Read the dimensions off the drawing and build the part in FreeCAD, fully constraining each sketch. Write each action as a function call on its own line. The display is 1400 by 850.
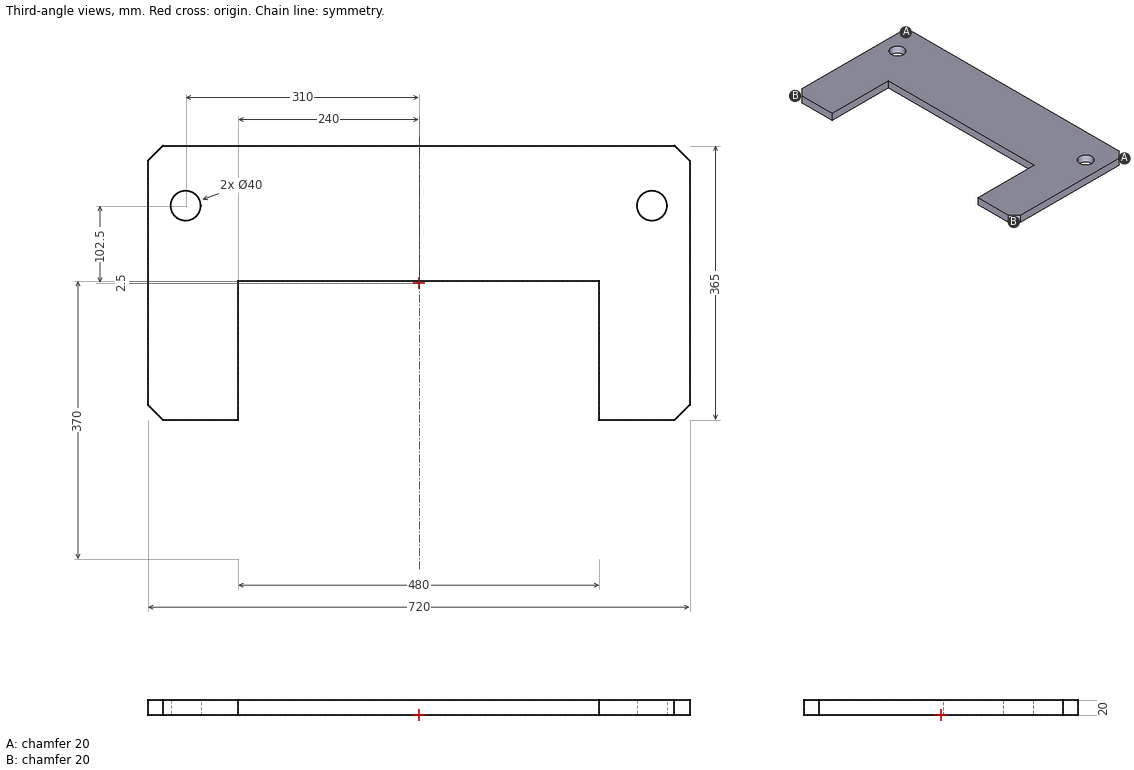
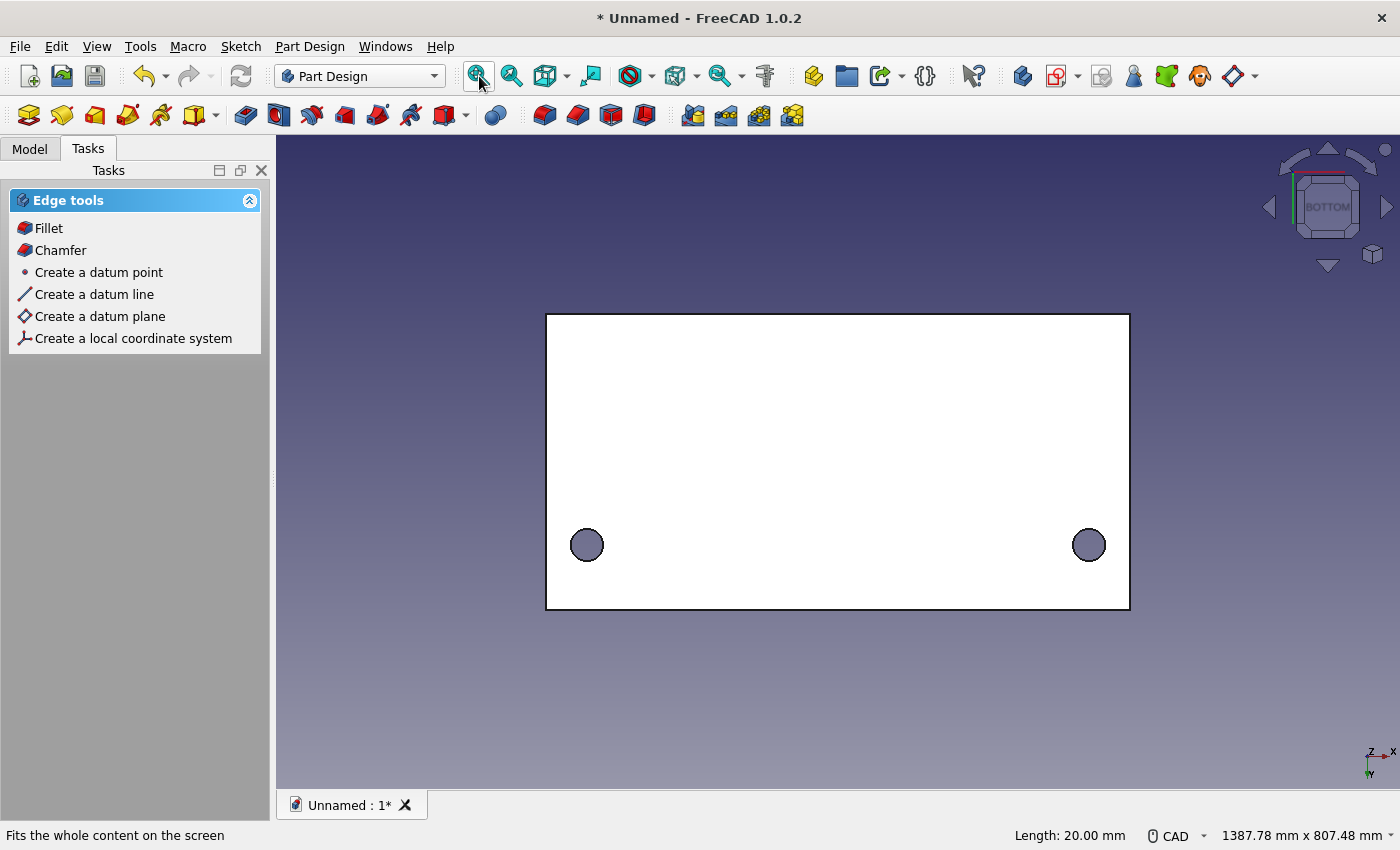
scroll(546, 609, up, 5)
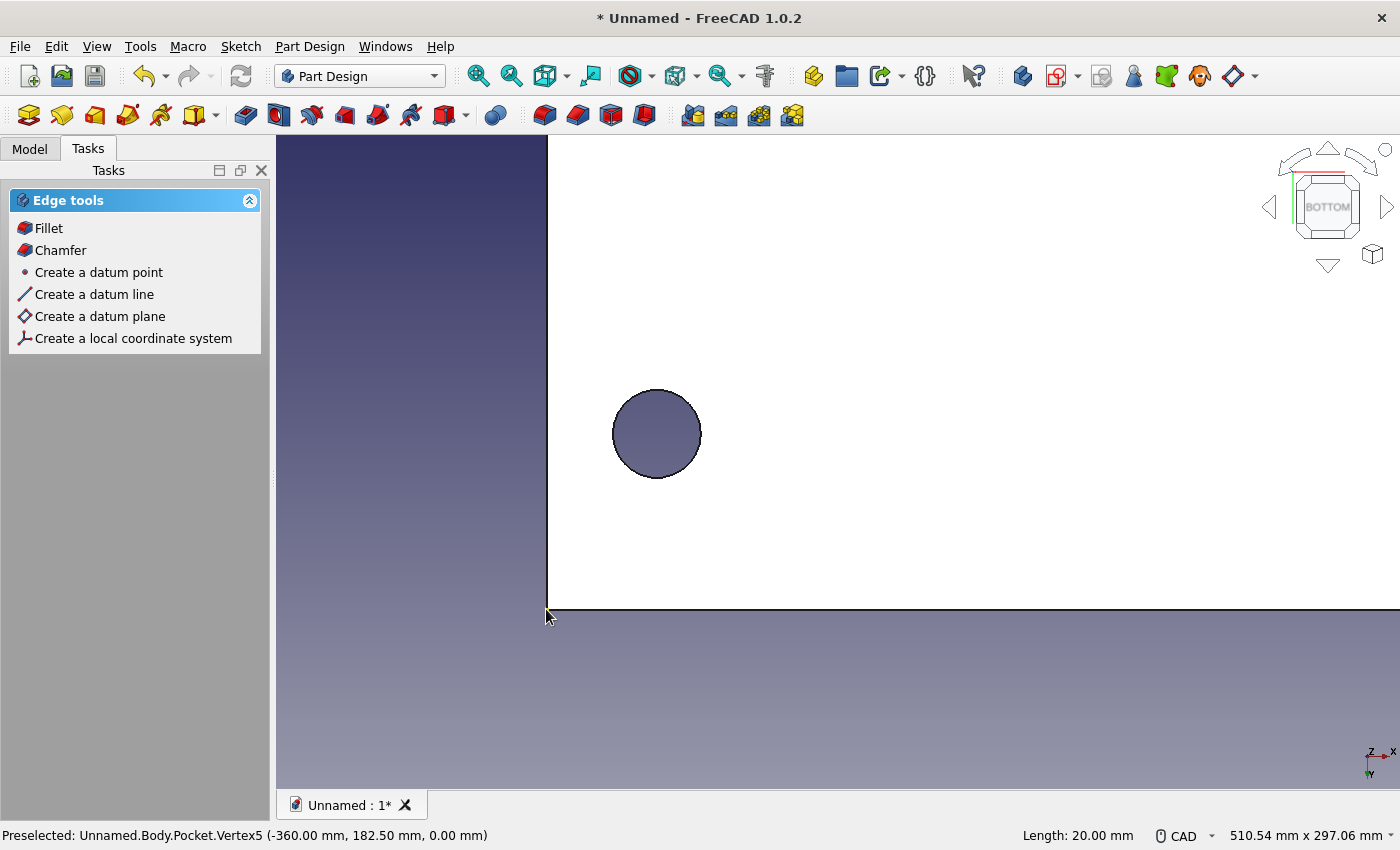
click(479, 76)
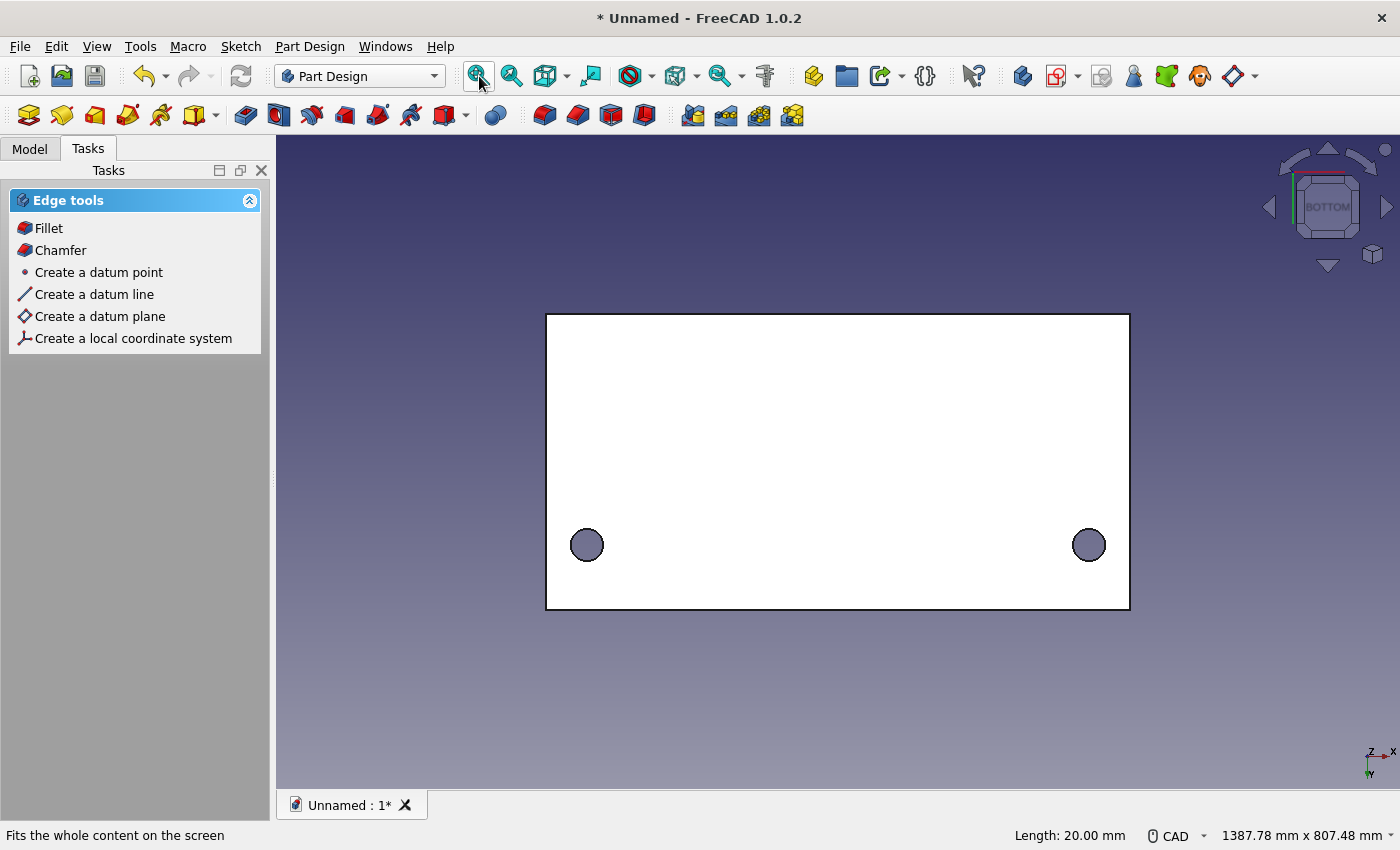
key(4)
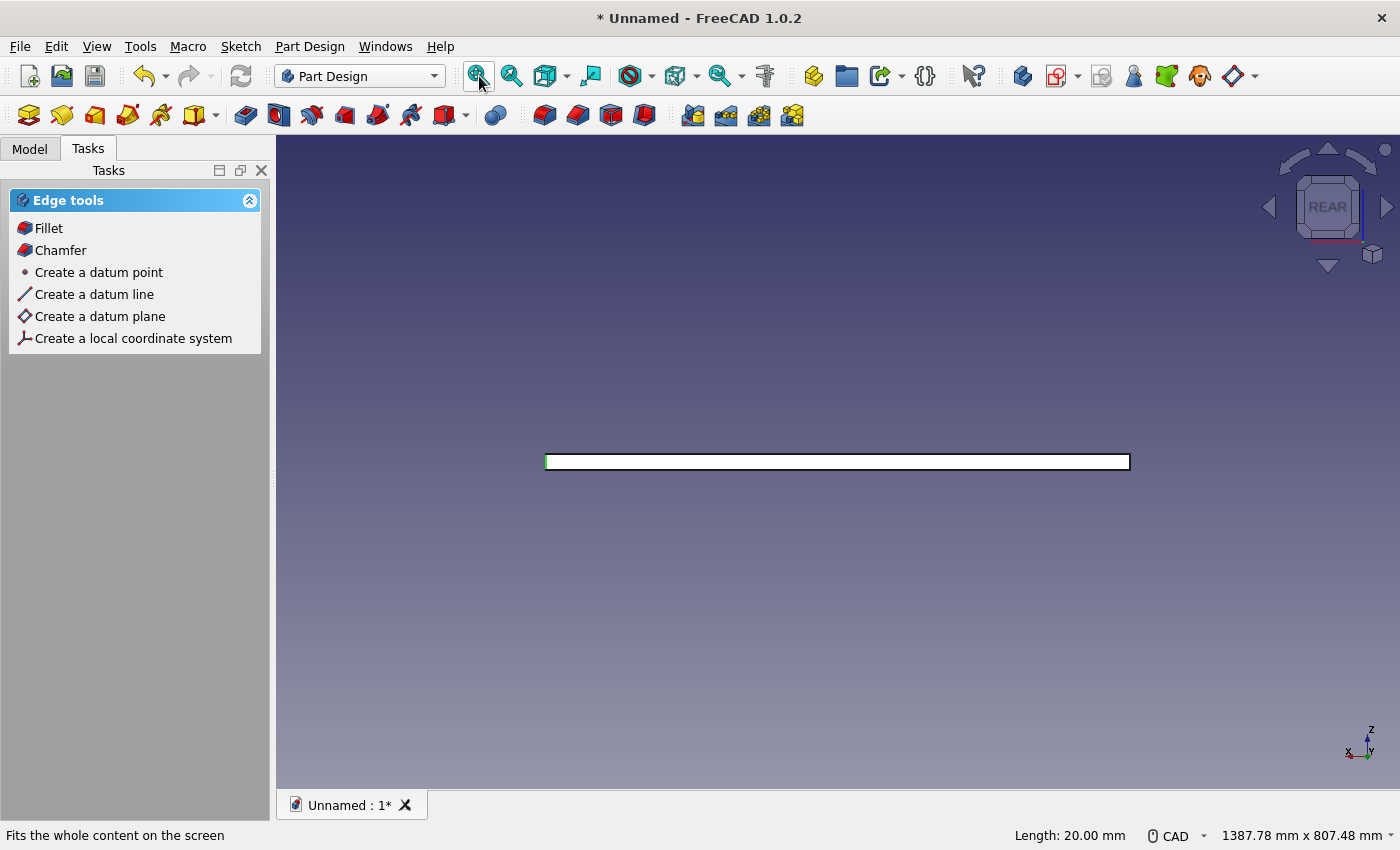
click(1130, 461, ctrl)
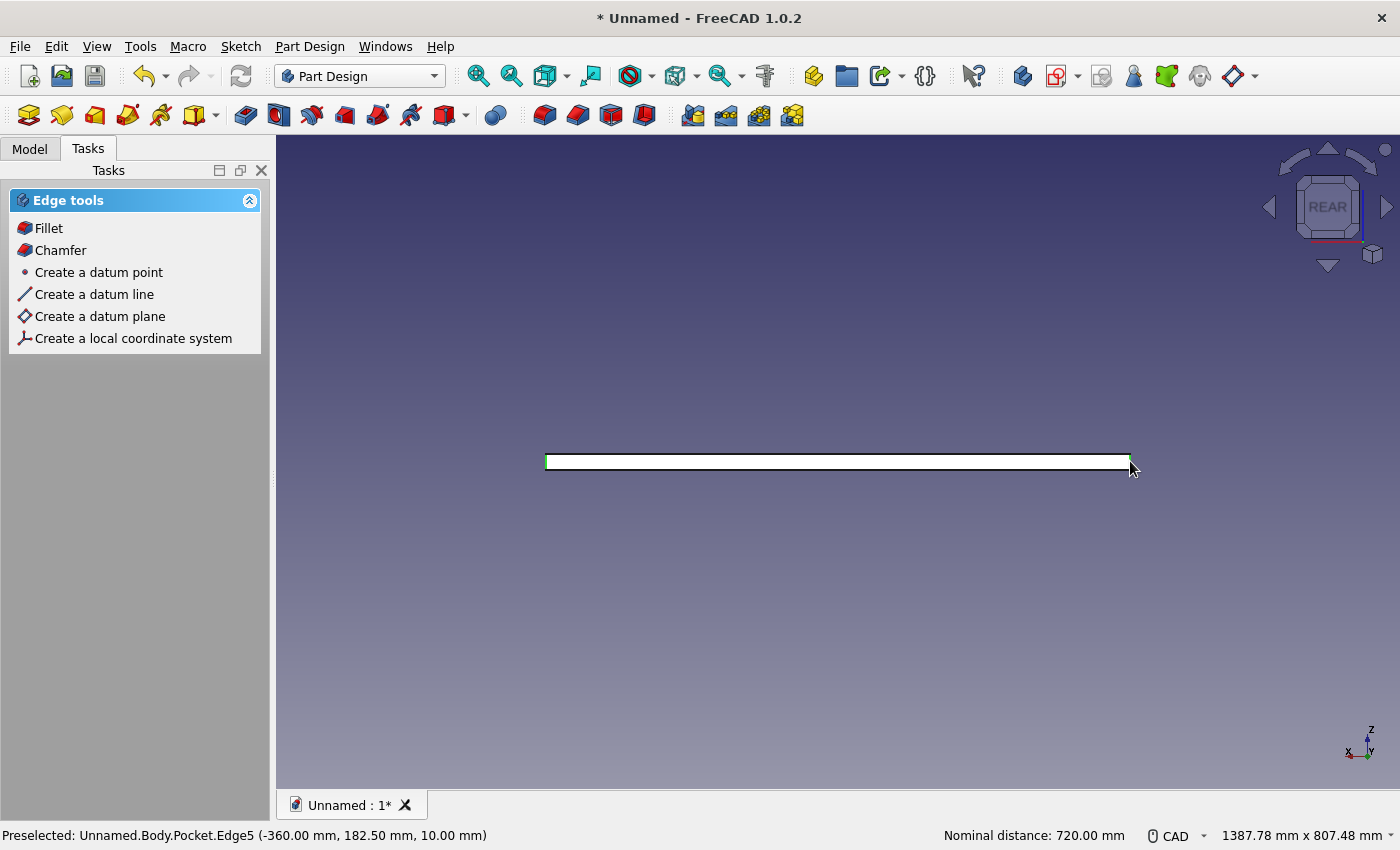
click(578, 116)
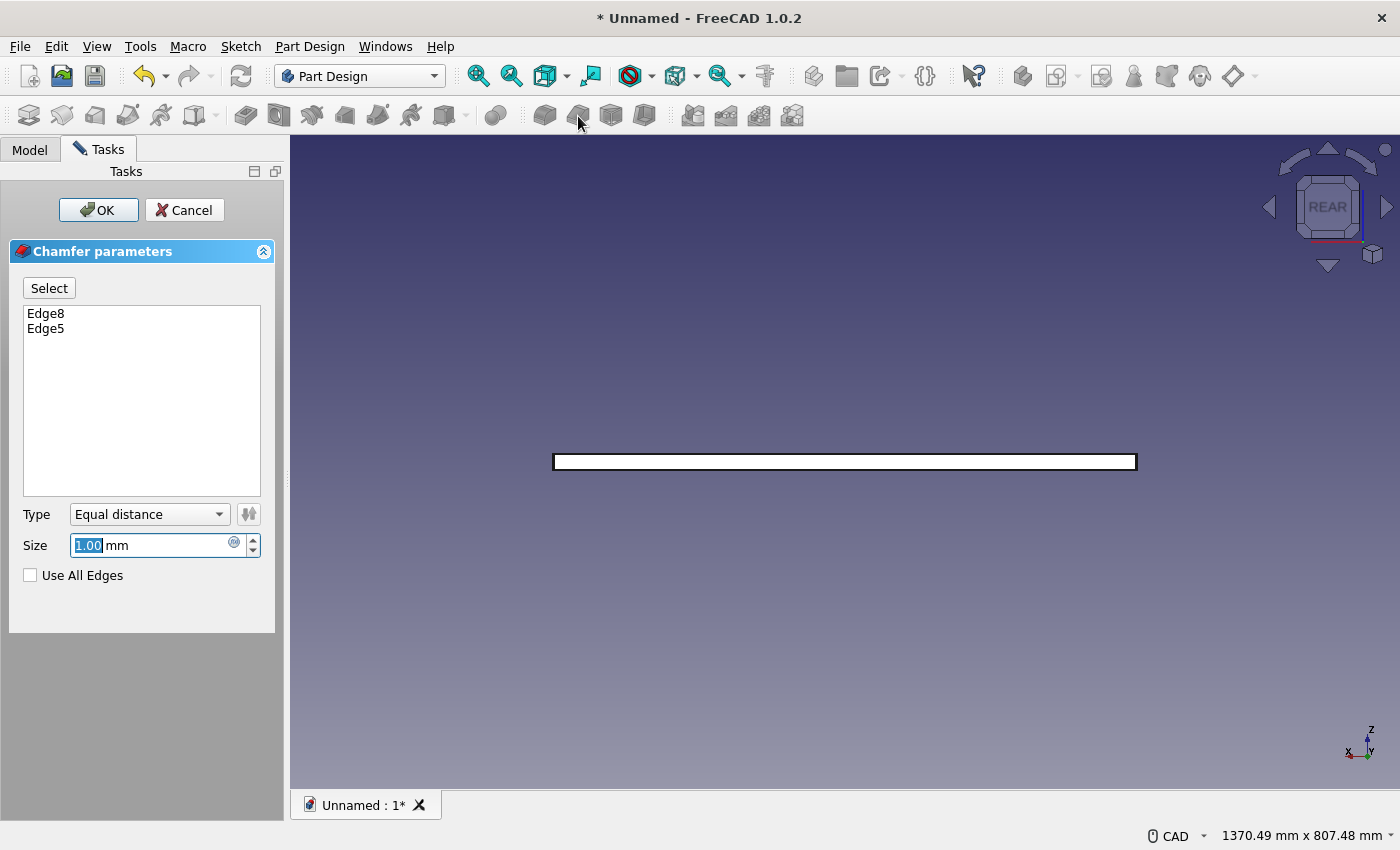
text(20)
key(Tab)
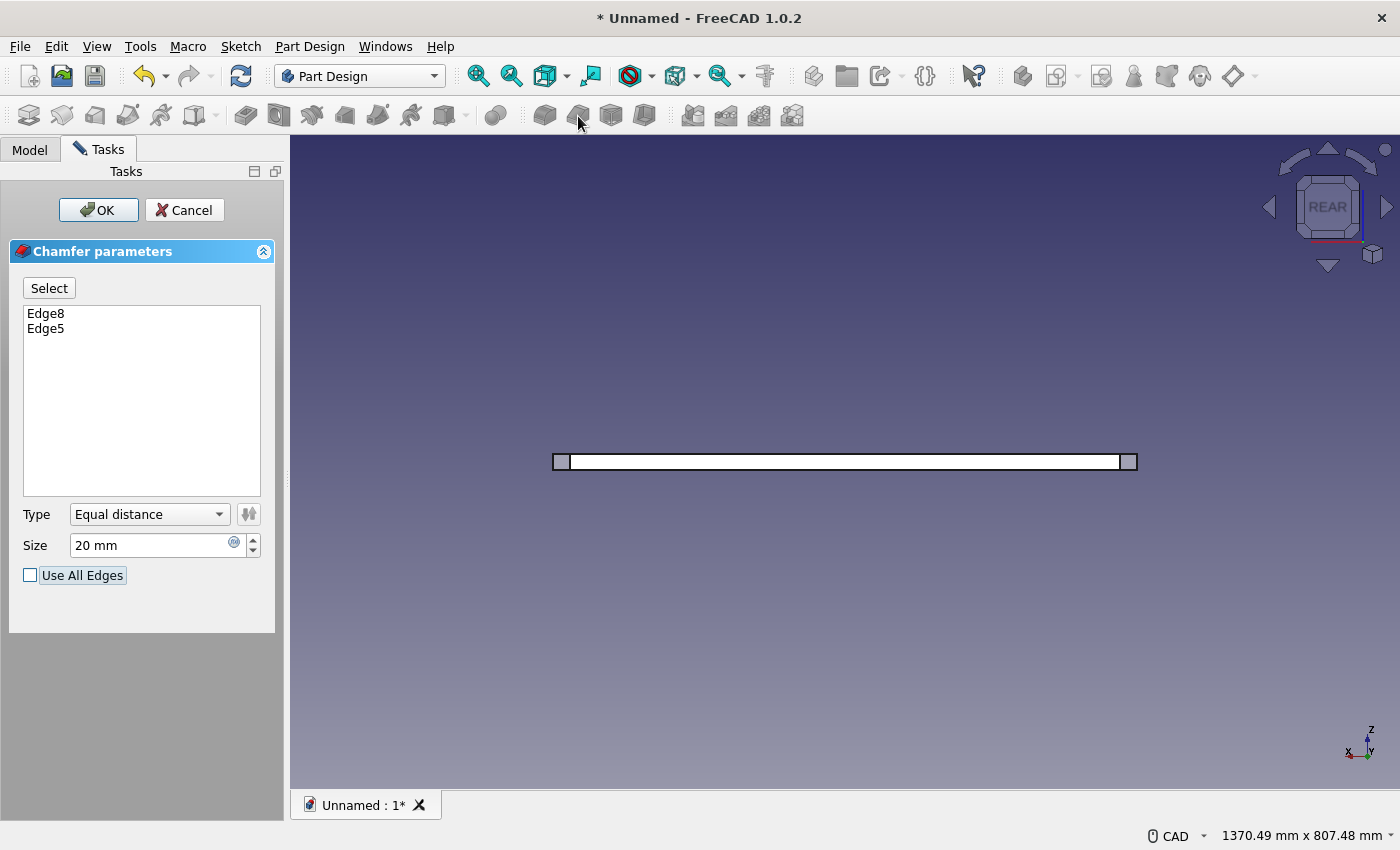
click(99, 210)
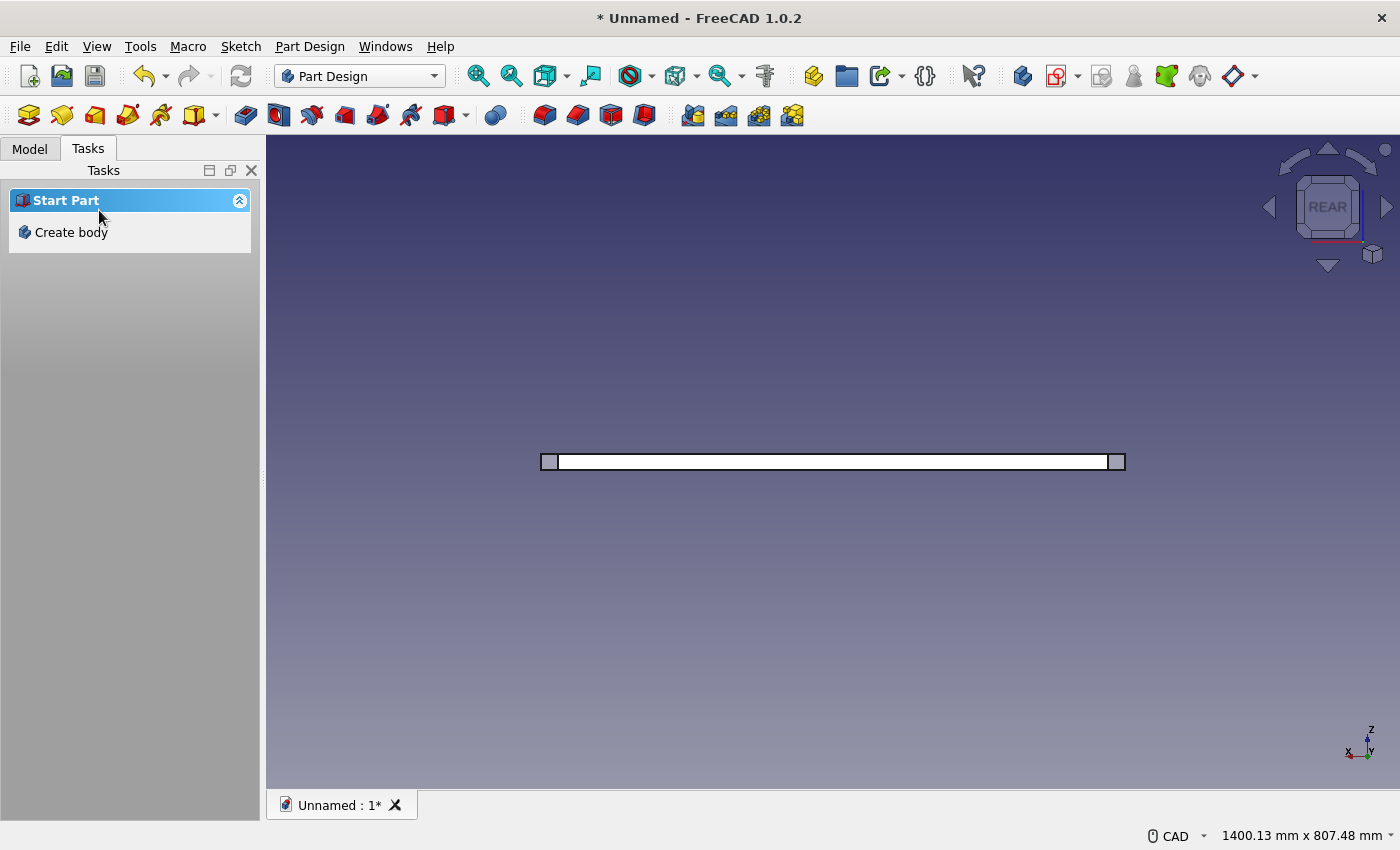
scroll(541, 461, up, 5)